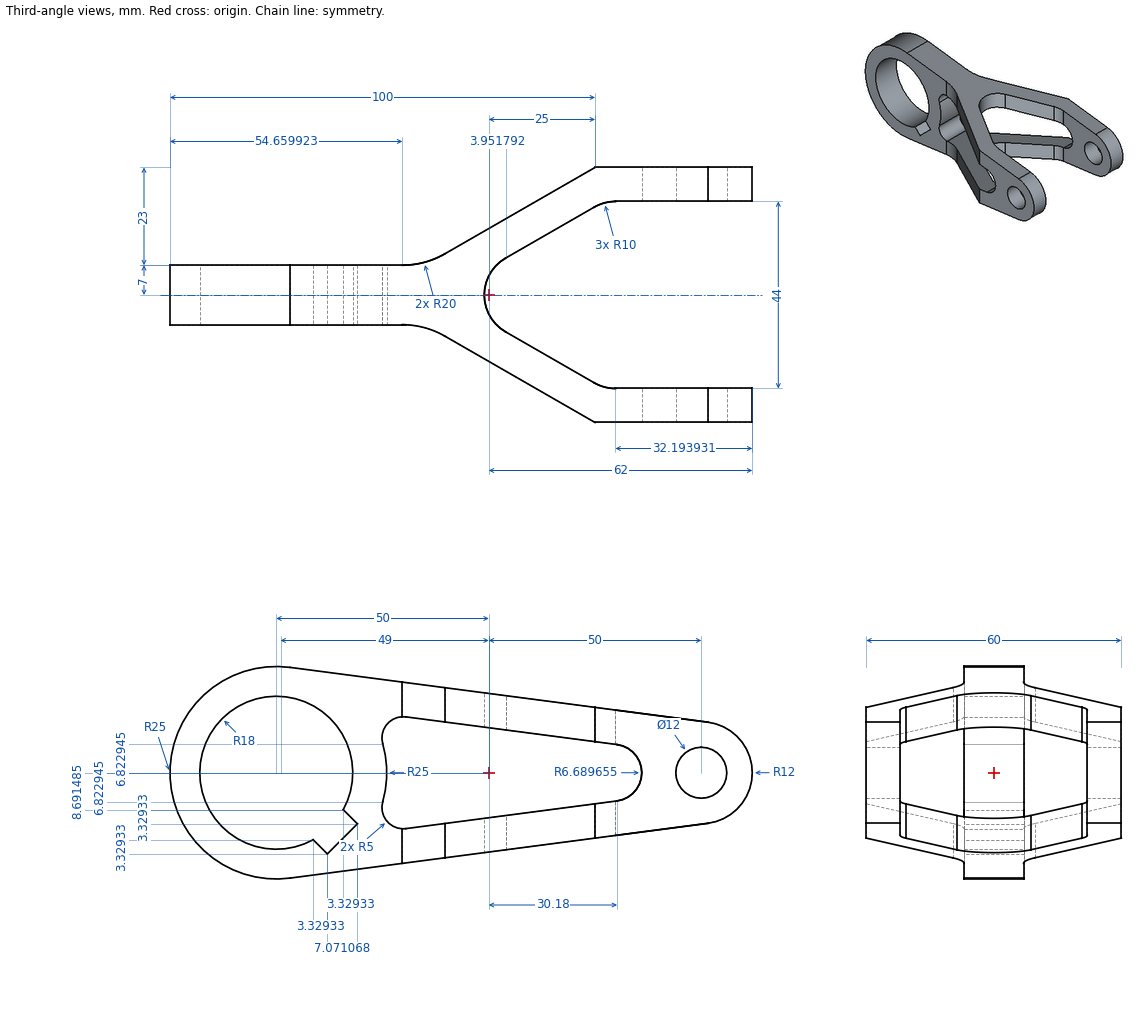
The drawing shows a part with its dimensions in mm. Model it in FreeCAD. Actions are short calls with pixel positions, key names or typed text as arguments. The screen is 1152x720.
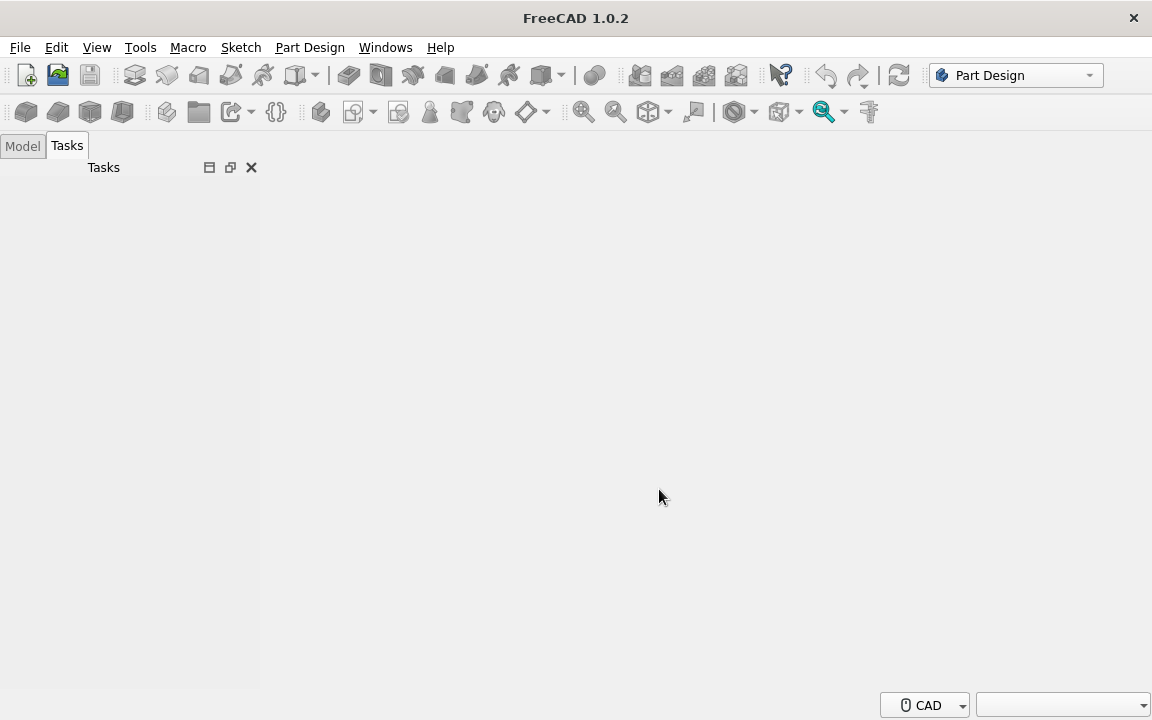
click(26, 76)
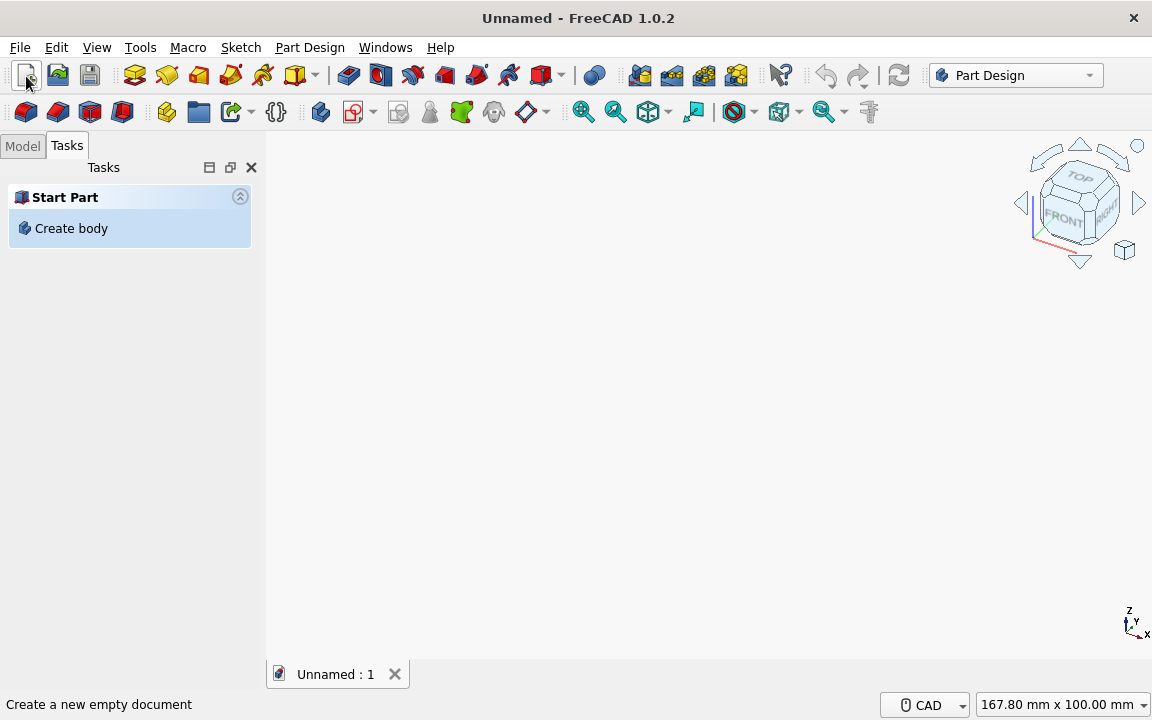
click(354, 112)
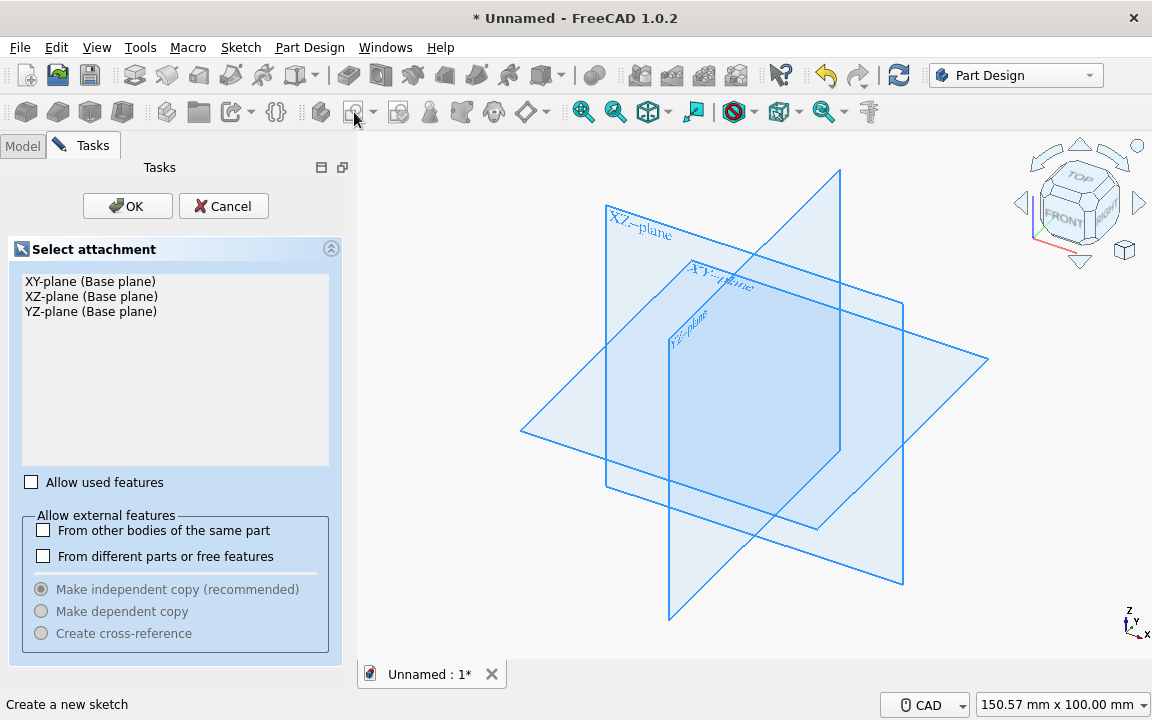
click(82, 296)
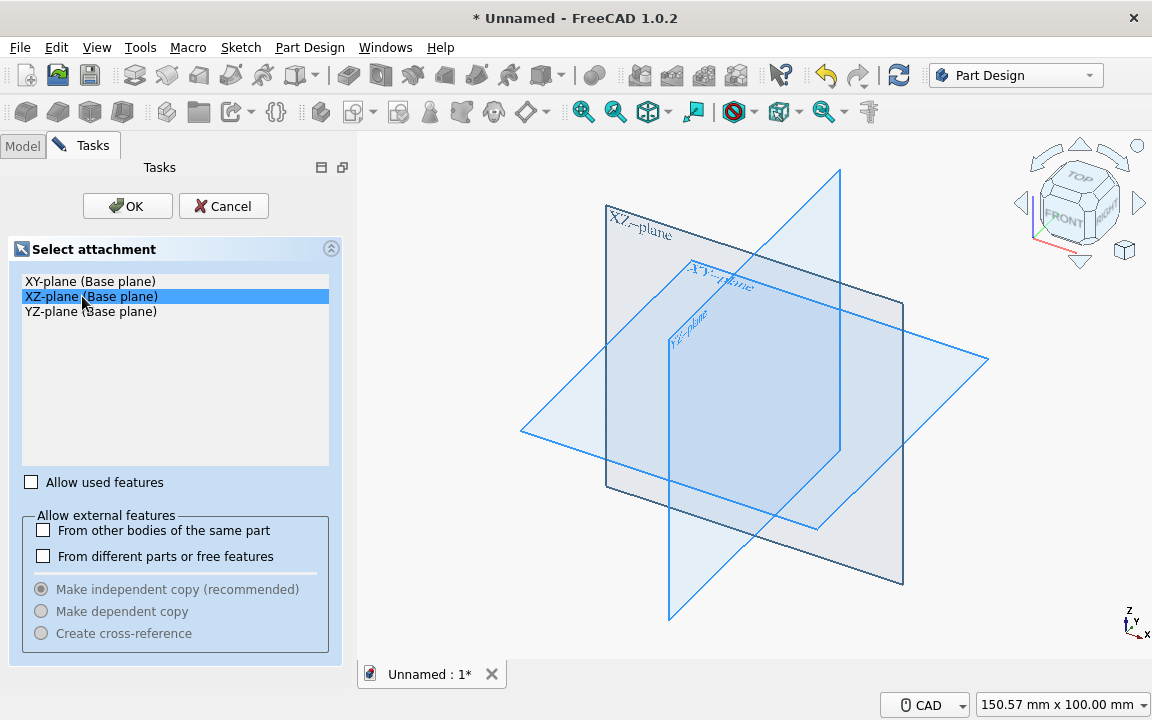
click(128, 206)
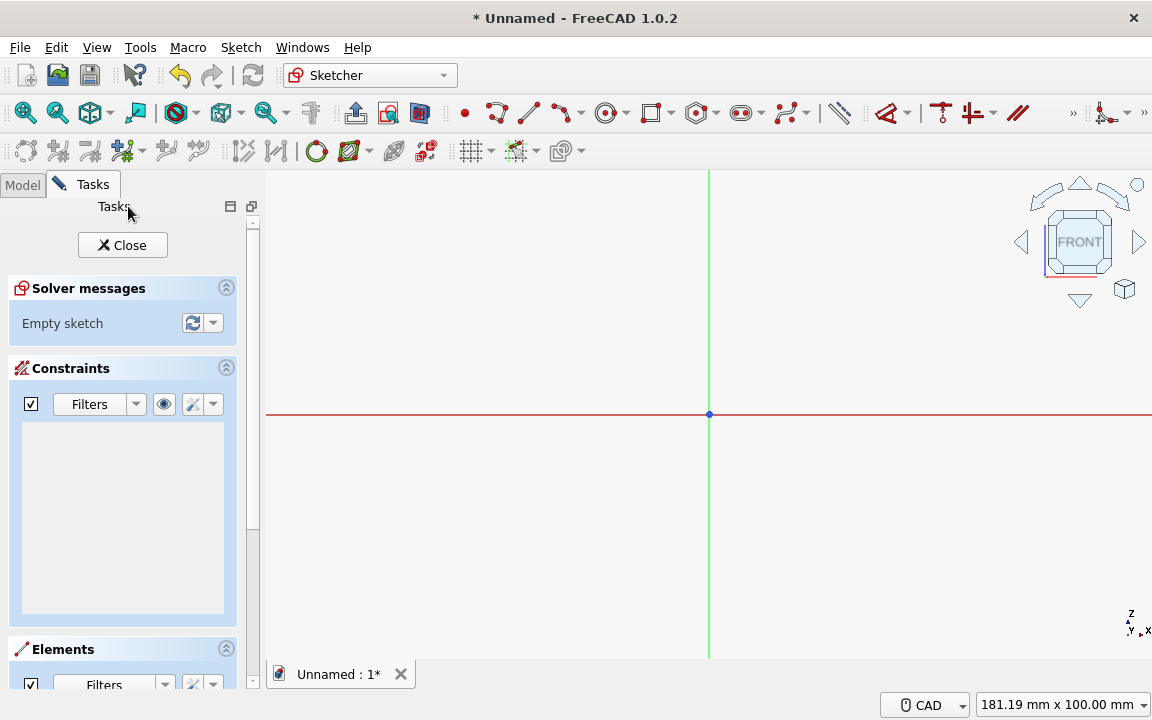
scroll(566, 414, down, 2)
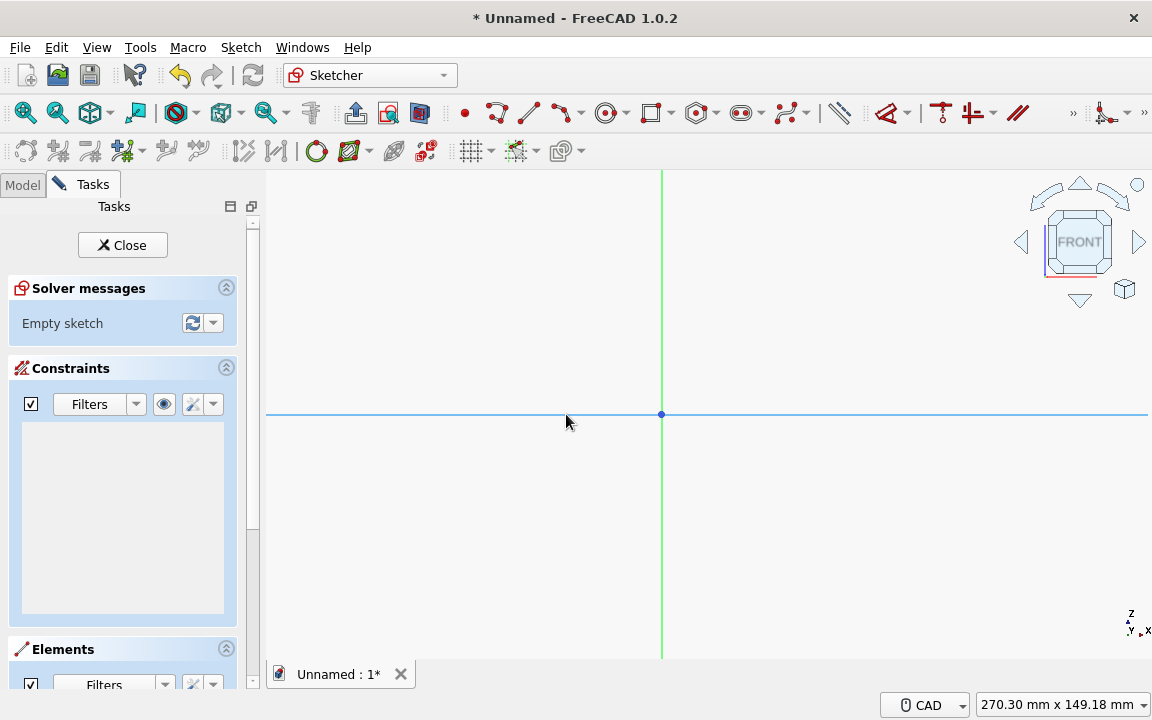
click(530, 114)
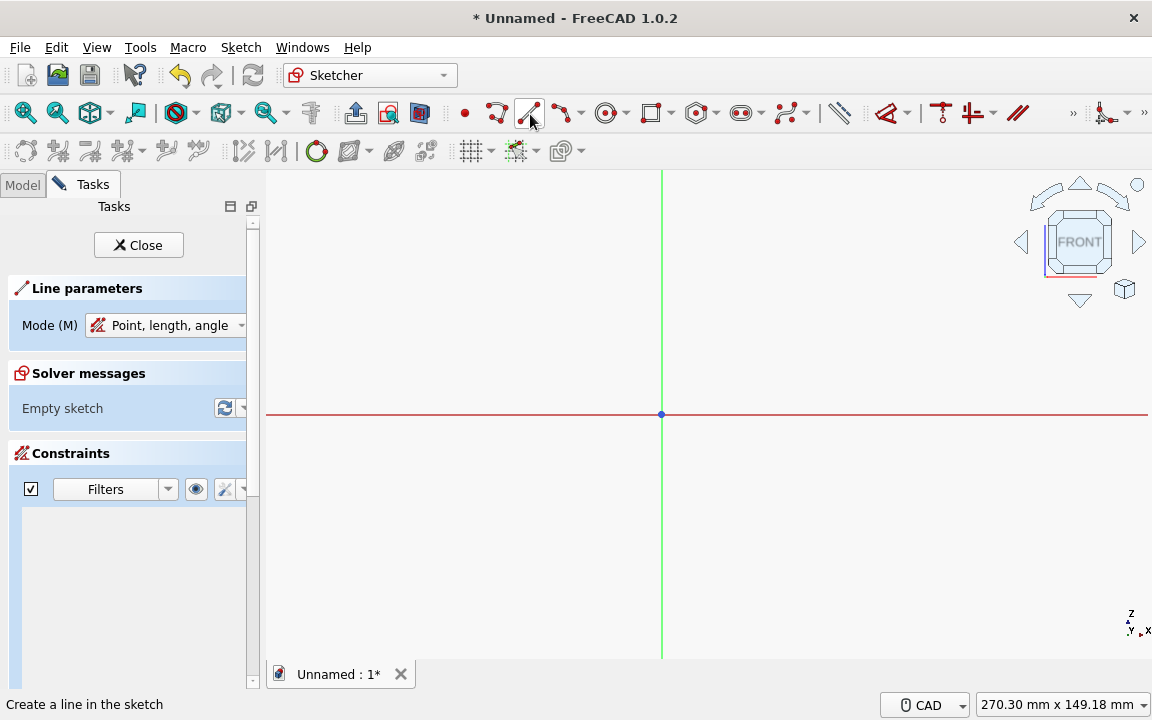
click(831, 454)
click(509, 496)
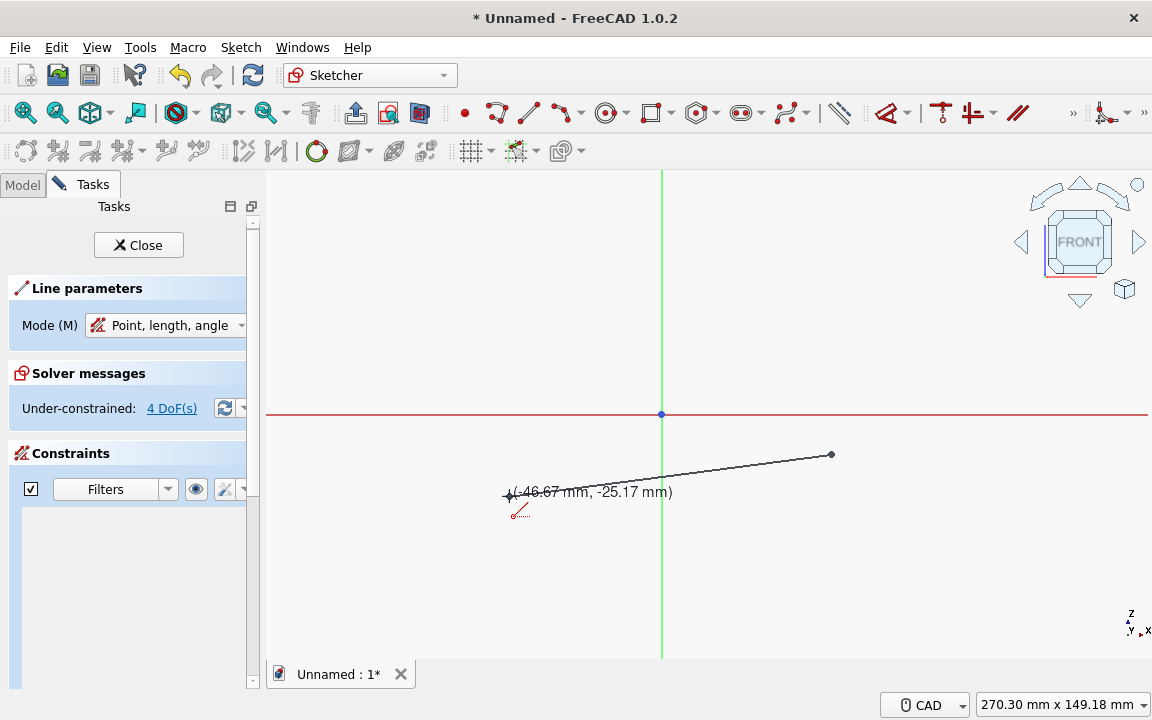
click(509, 333)
click(831, 375)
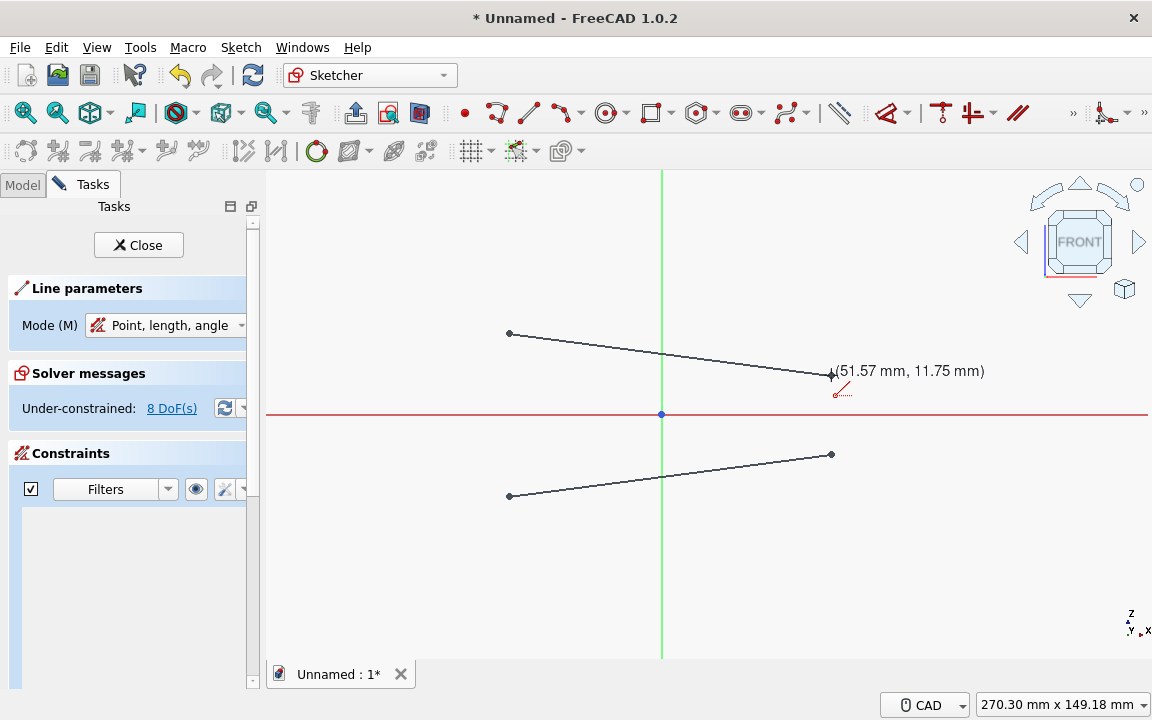
click(562, 114)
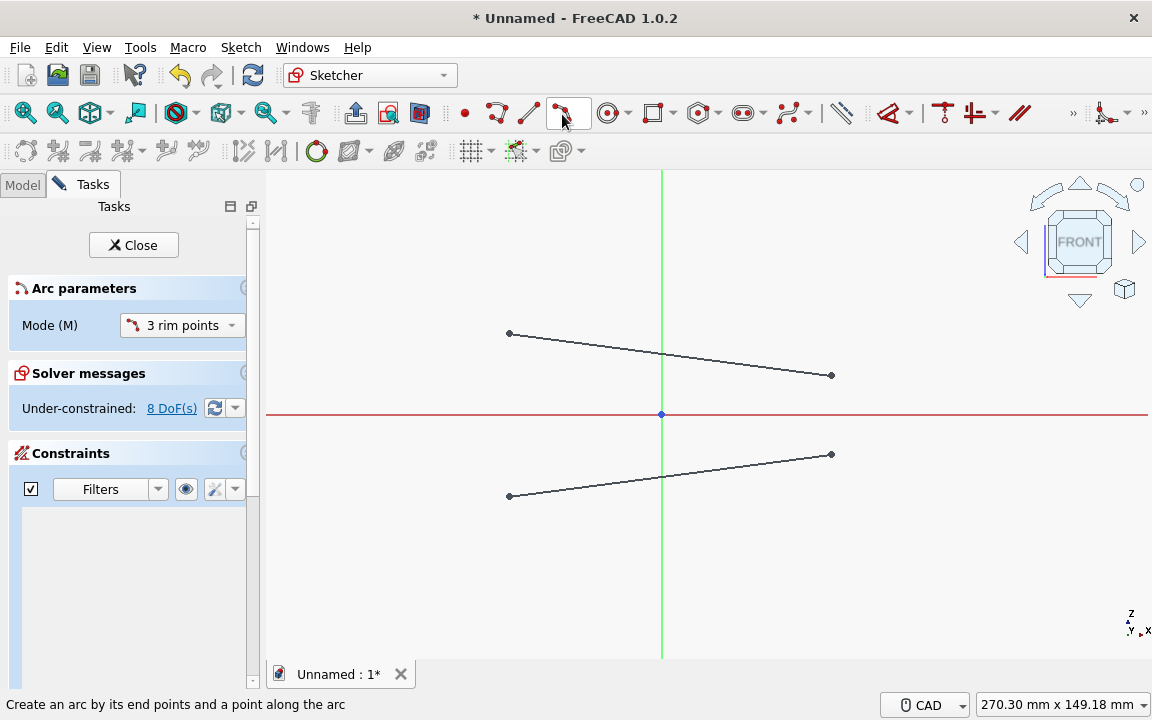
click(509, 497)
click(509, 334)
click(421, 387)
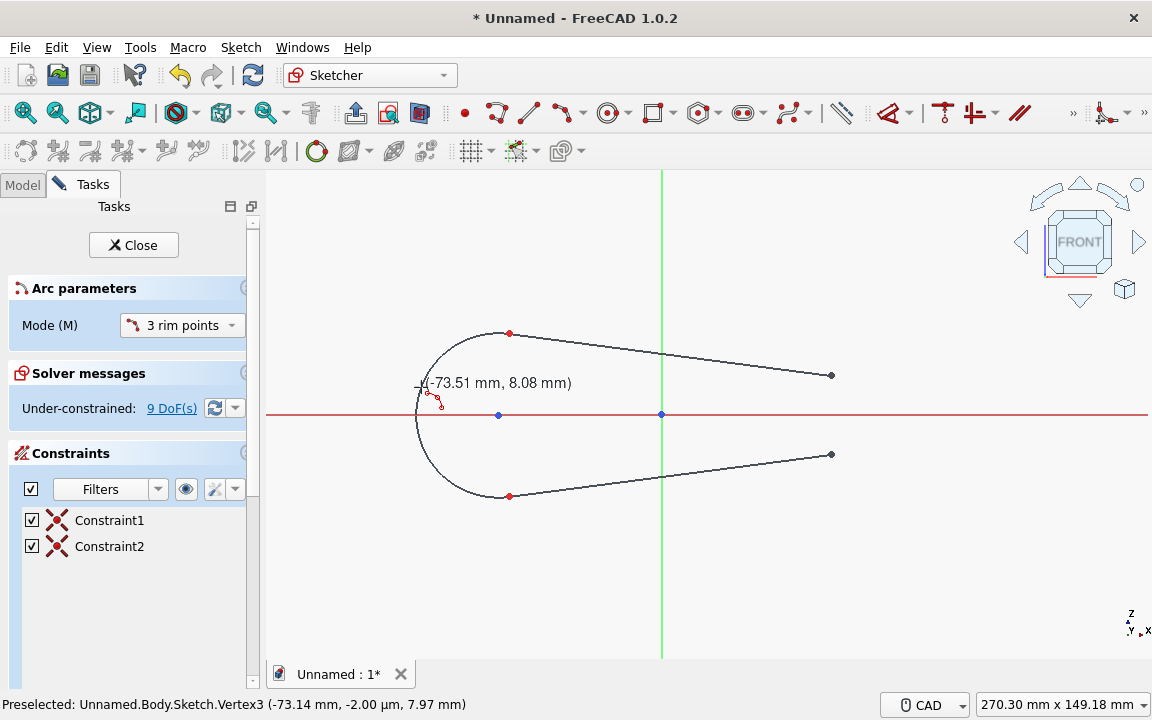
click(831, 376)
click(831, 455)
click(859, 436)
key(Escape)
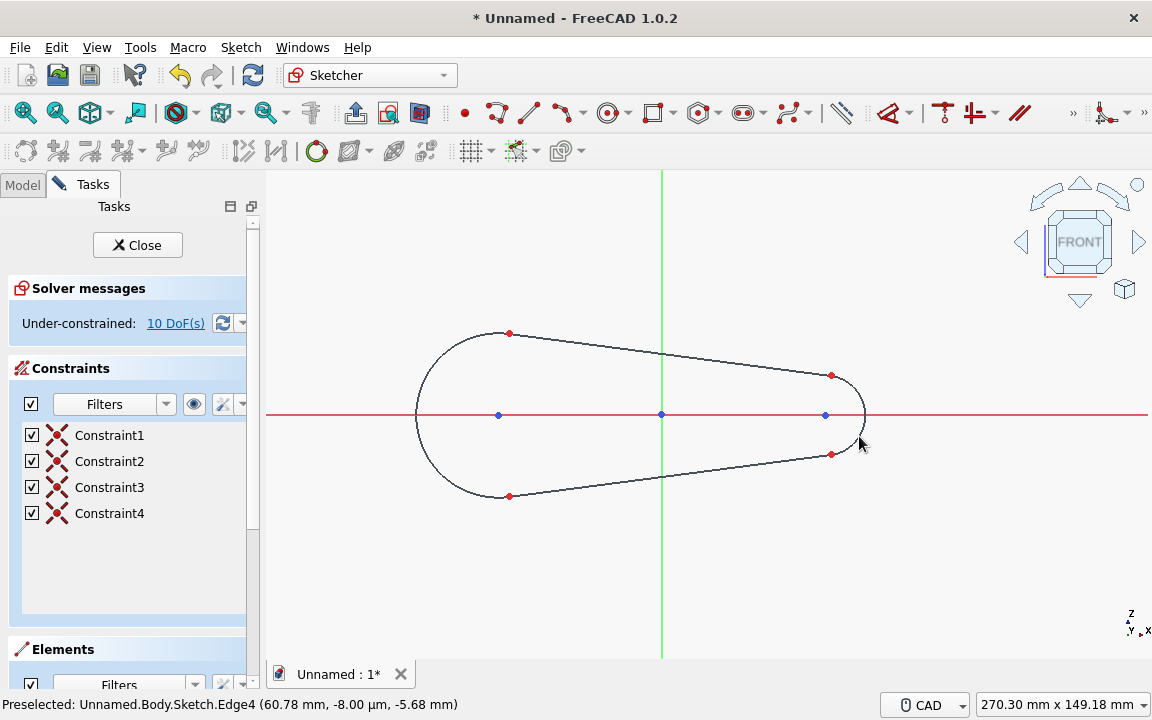
click(734, 468)